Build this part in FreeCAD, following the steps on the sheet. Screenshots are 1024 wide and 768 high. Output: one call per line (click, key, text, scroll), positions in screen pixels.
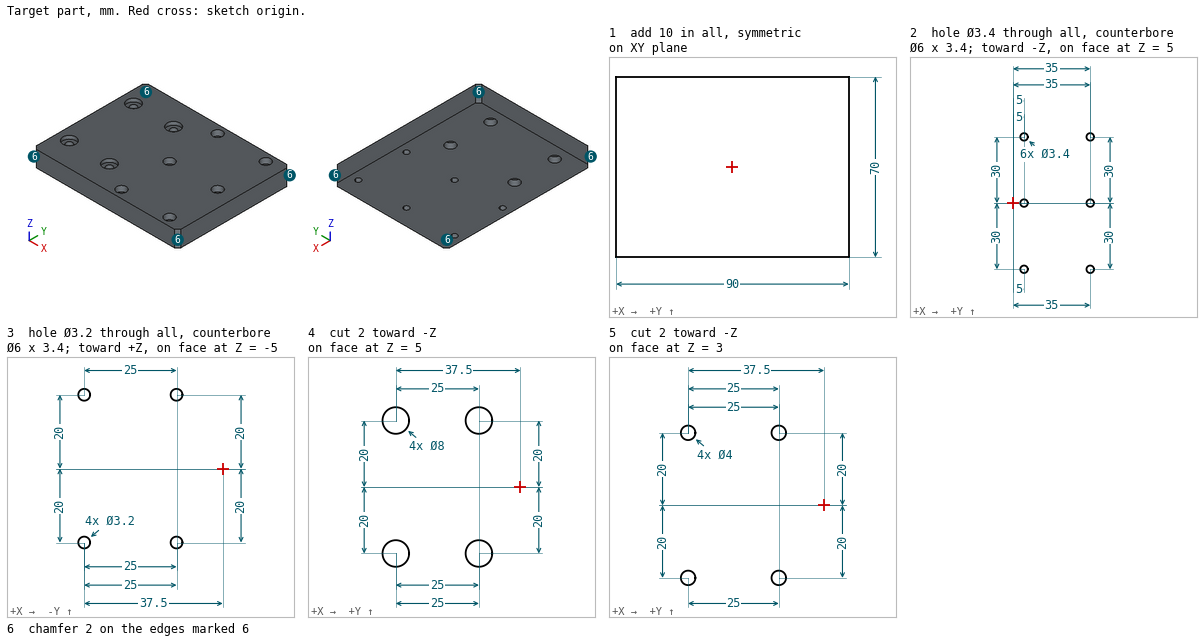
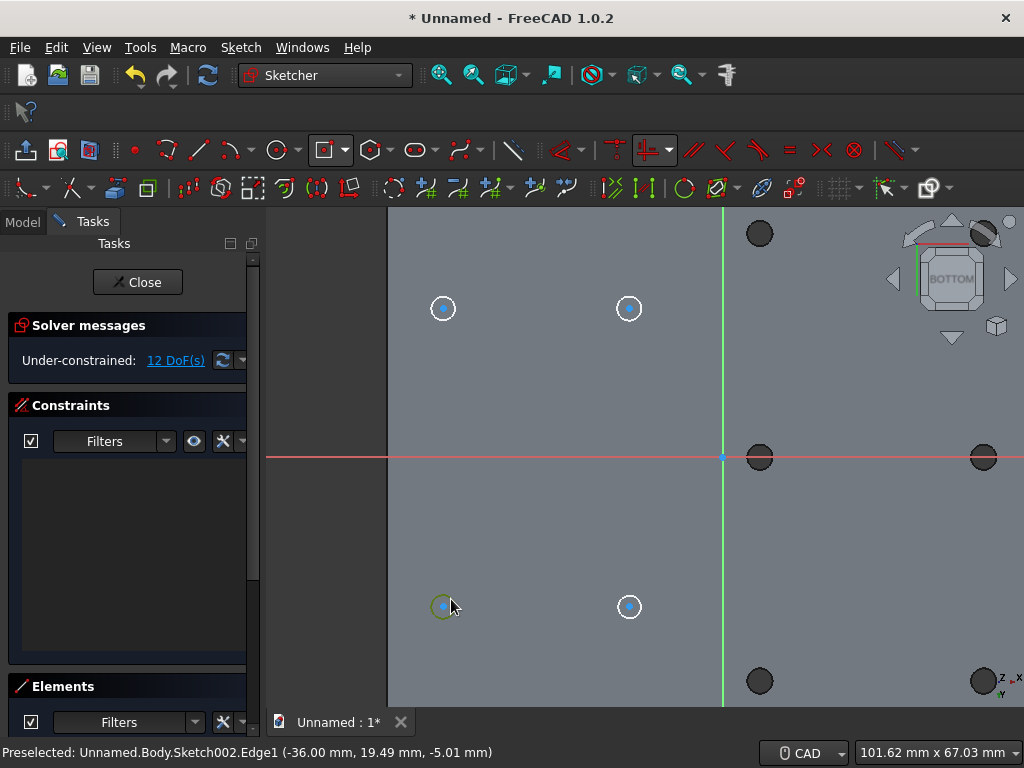
scroll(638, 599, up, 2)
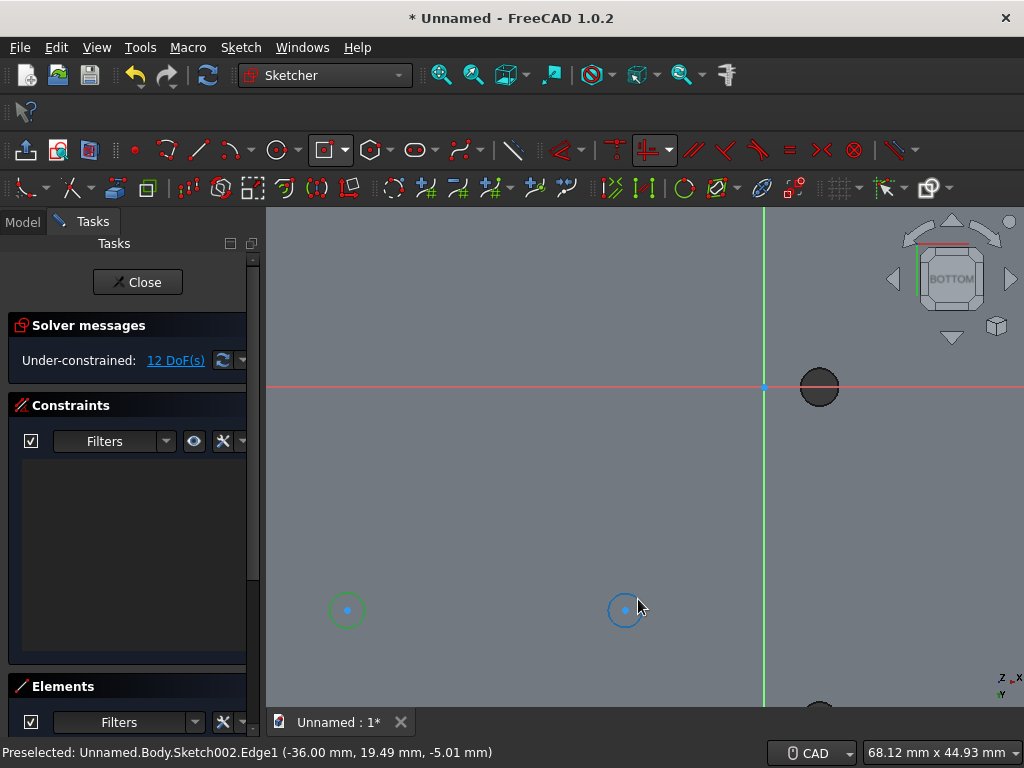
click(637, 599)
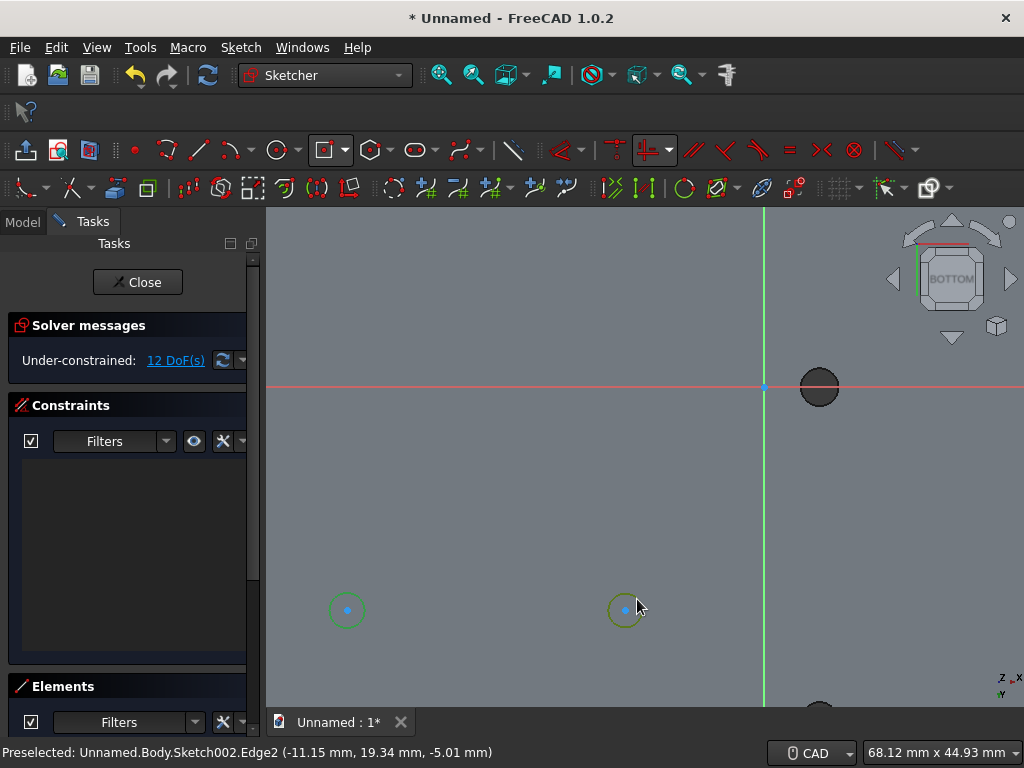
scroll(638, 599, down, 2)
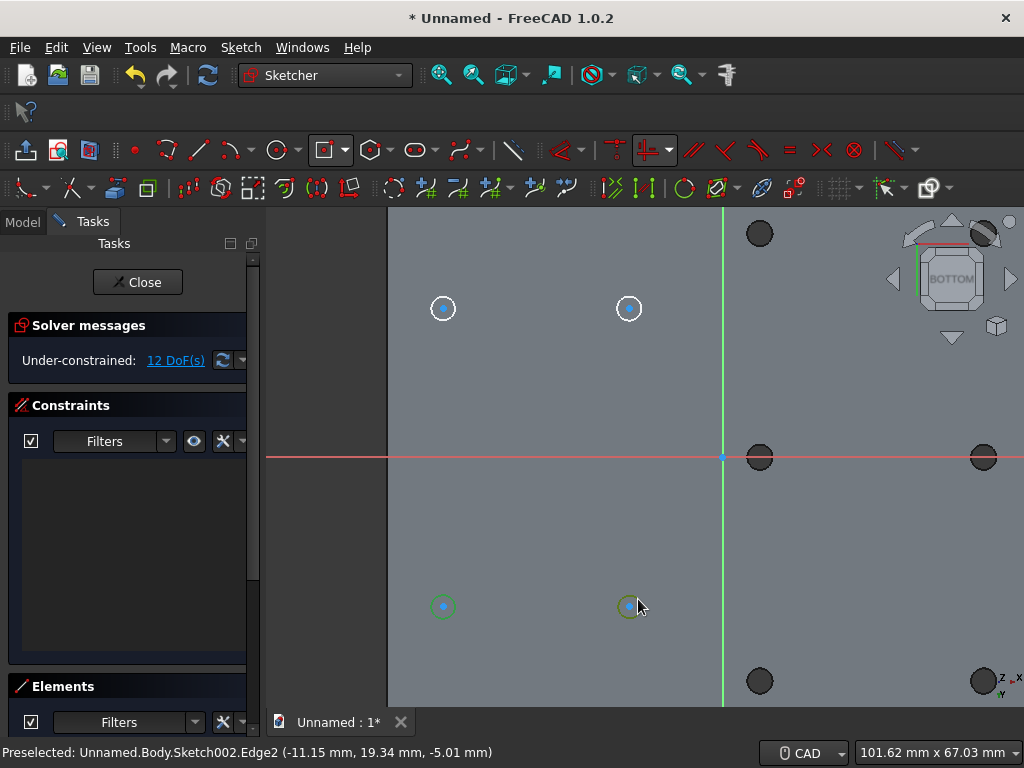
click(638, 300)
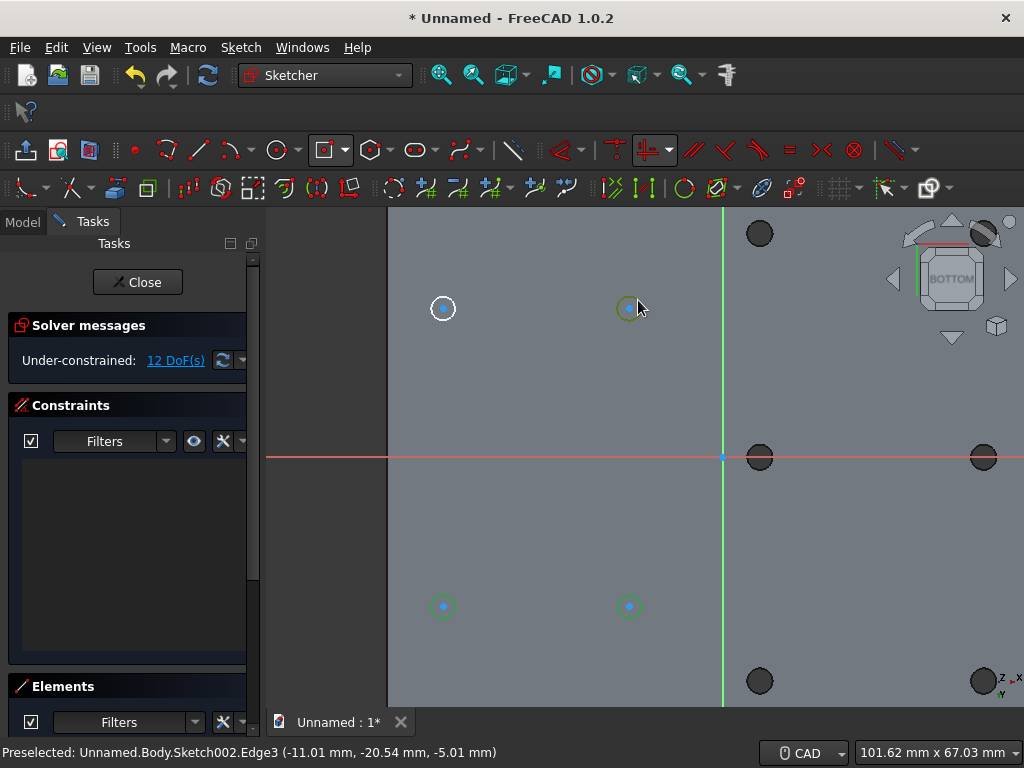
click(451, 300)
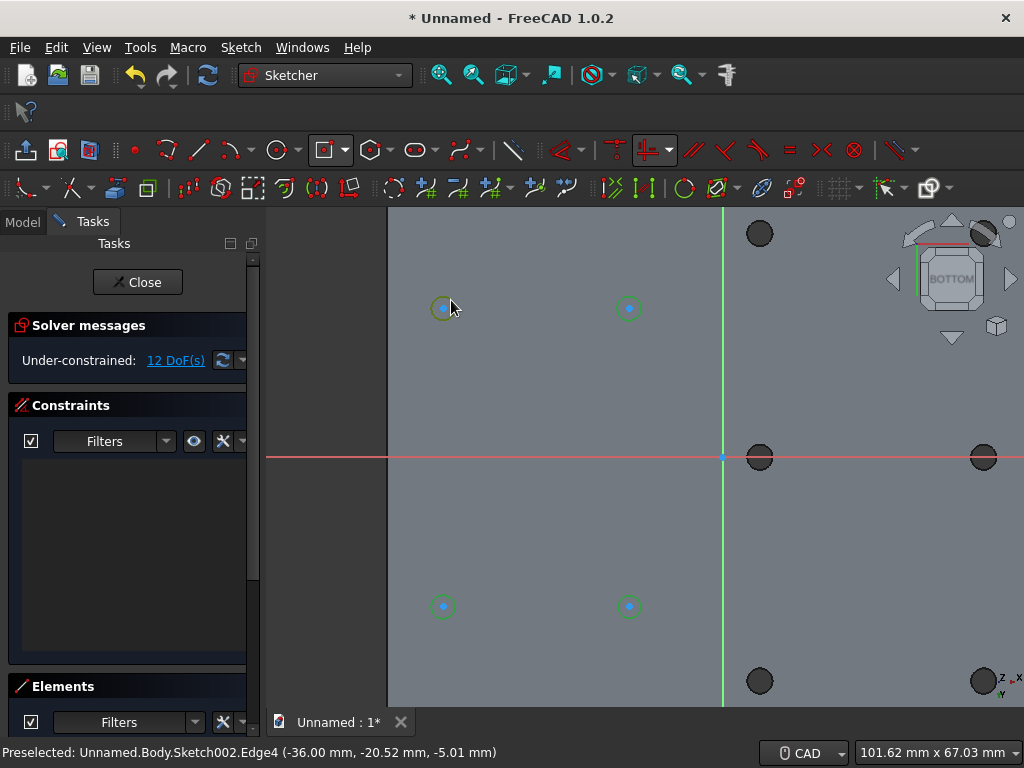
click(790, 150)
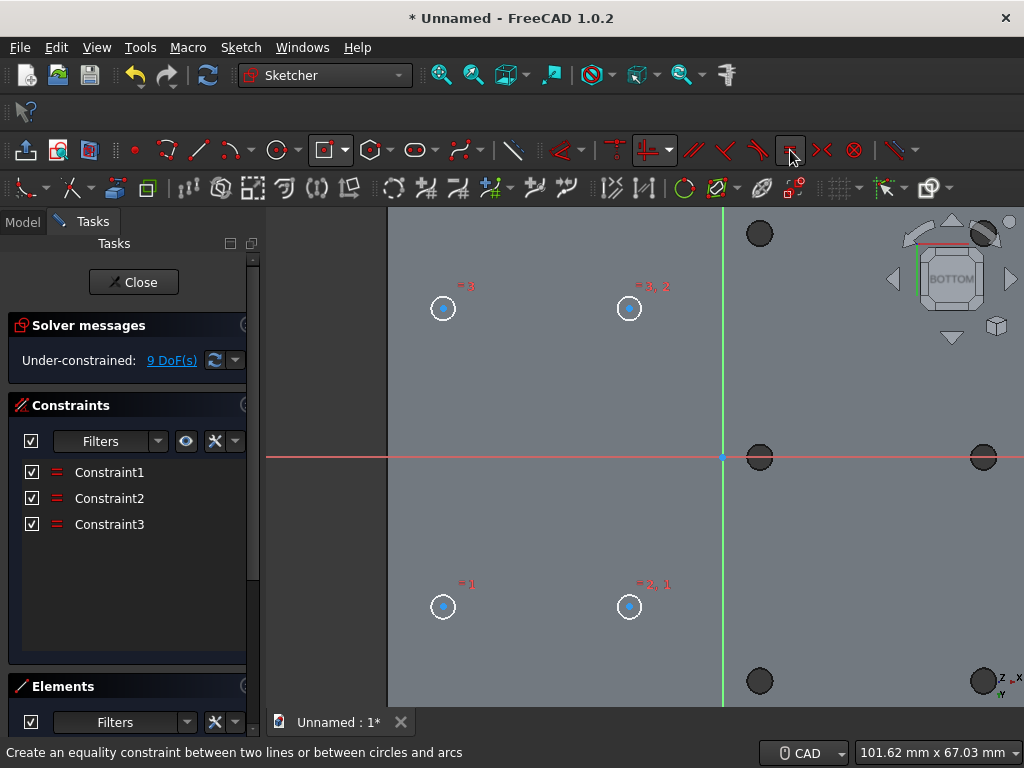
click(560, 150)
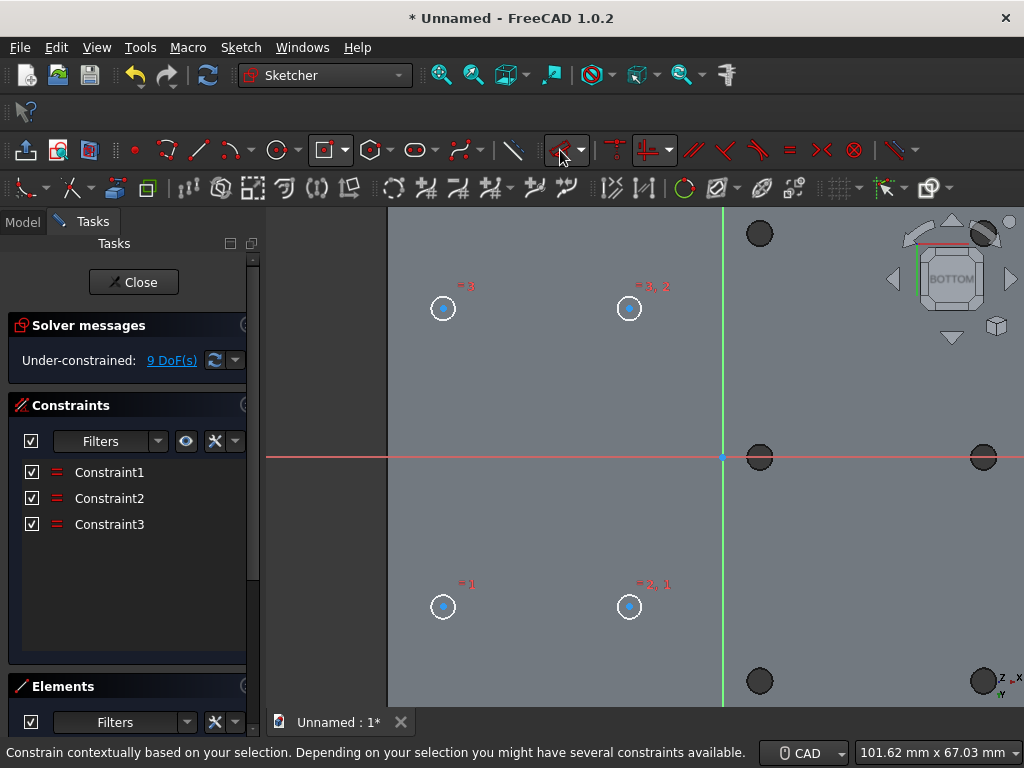
scroll(451, 599, up, 3)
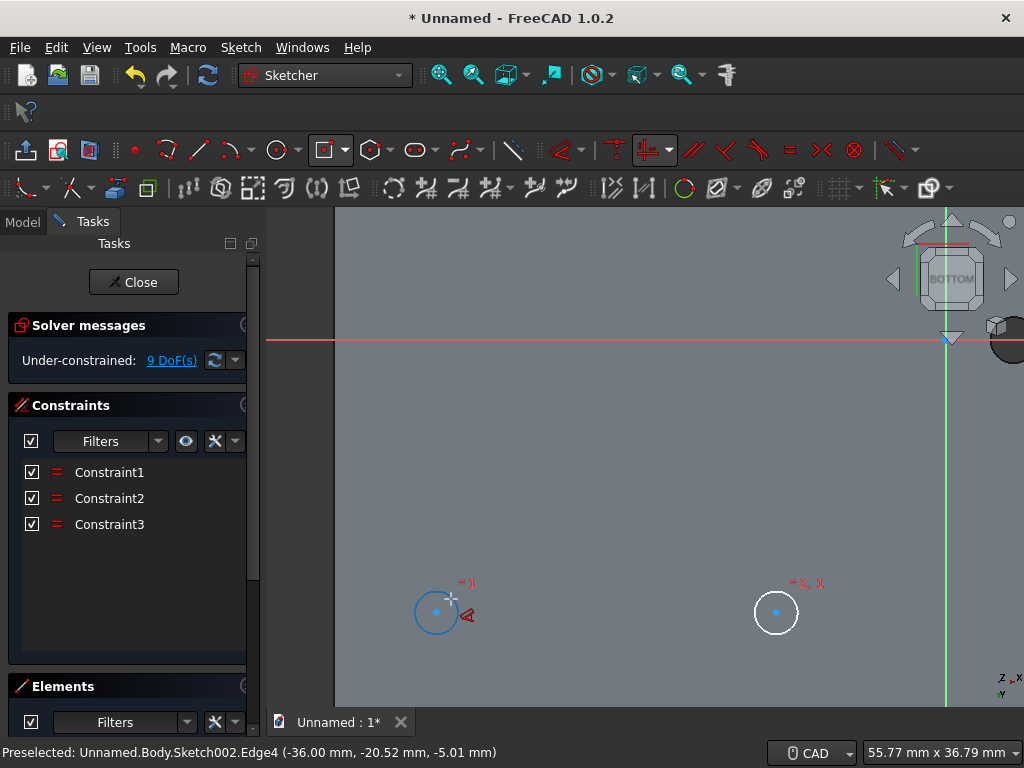
click(452, 598)
click(475, 576)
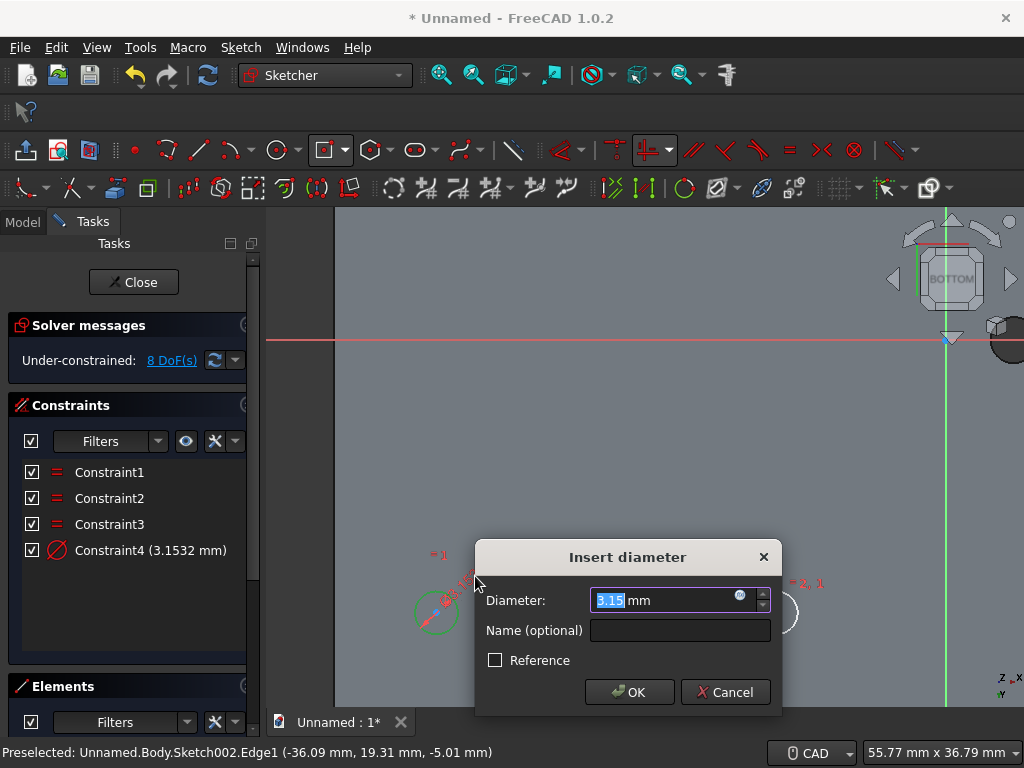
text(3.2)
key(Return)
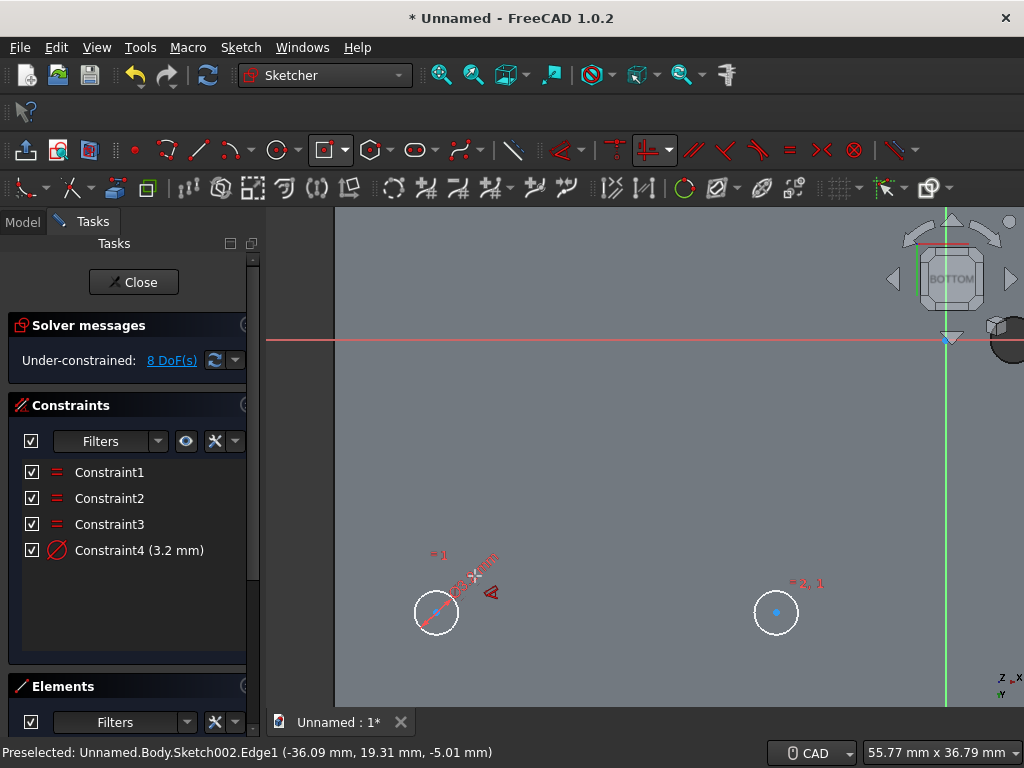
click(436, 613)
click(402, 477)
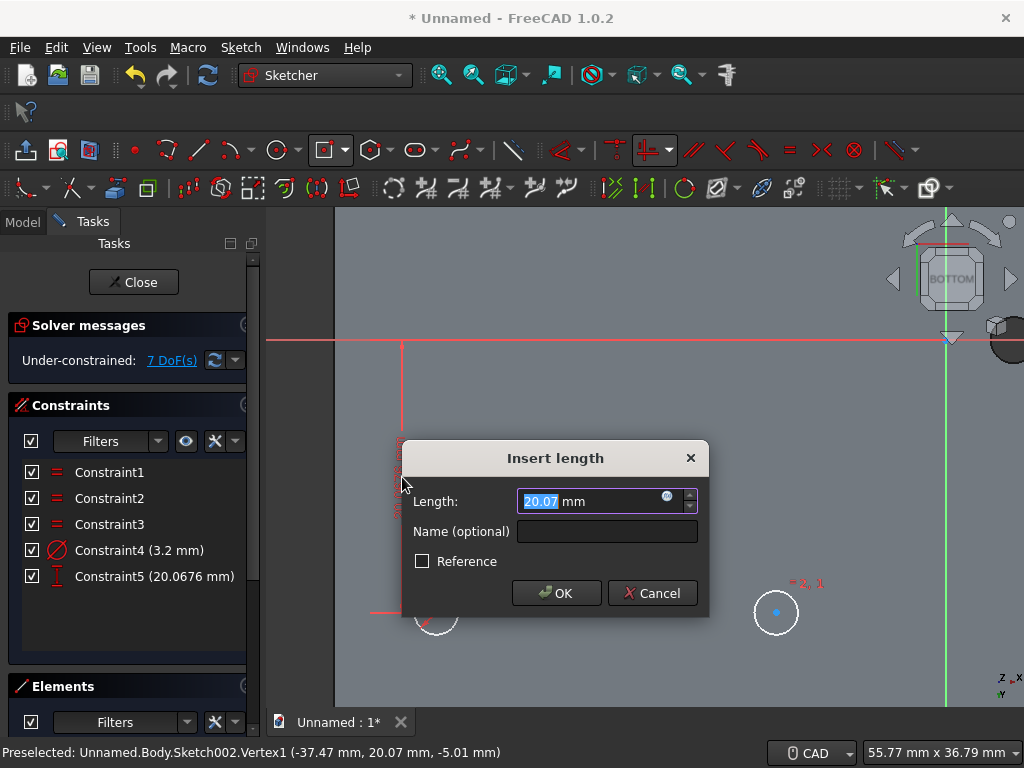
text(20)
key(Return)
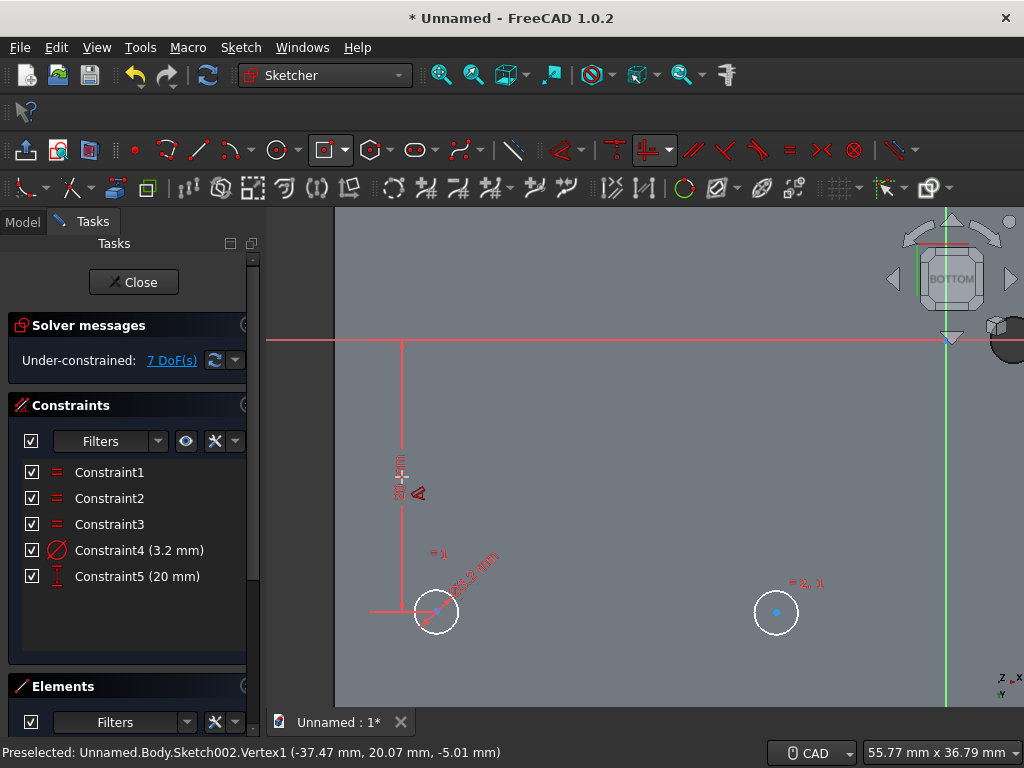
click(776, 613)
click(742, 477)